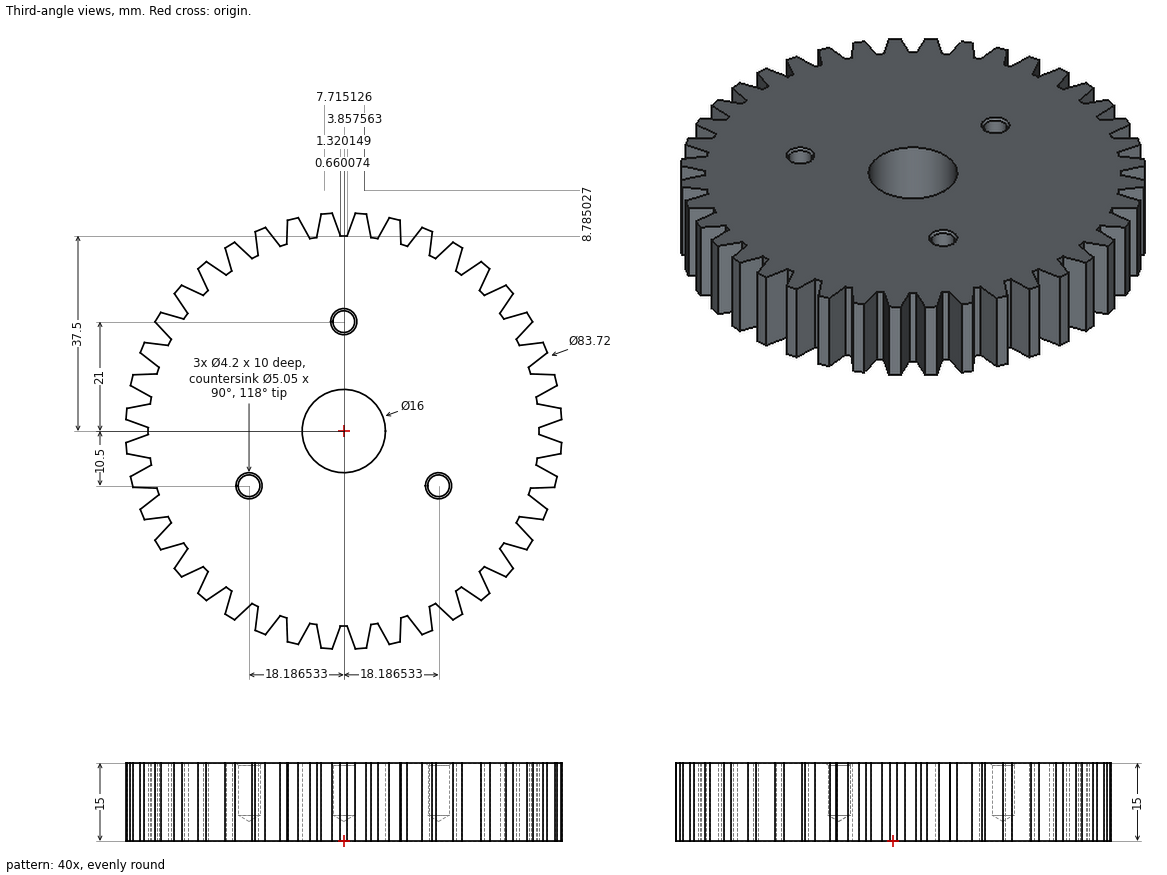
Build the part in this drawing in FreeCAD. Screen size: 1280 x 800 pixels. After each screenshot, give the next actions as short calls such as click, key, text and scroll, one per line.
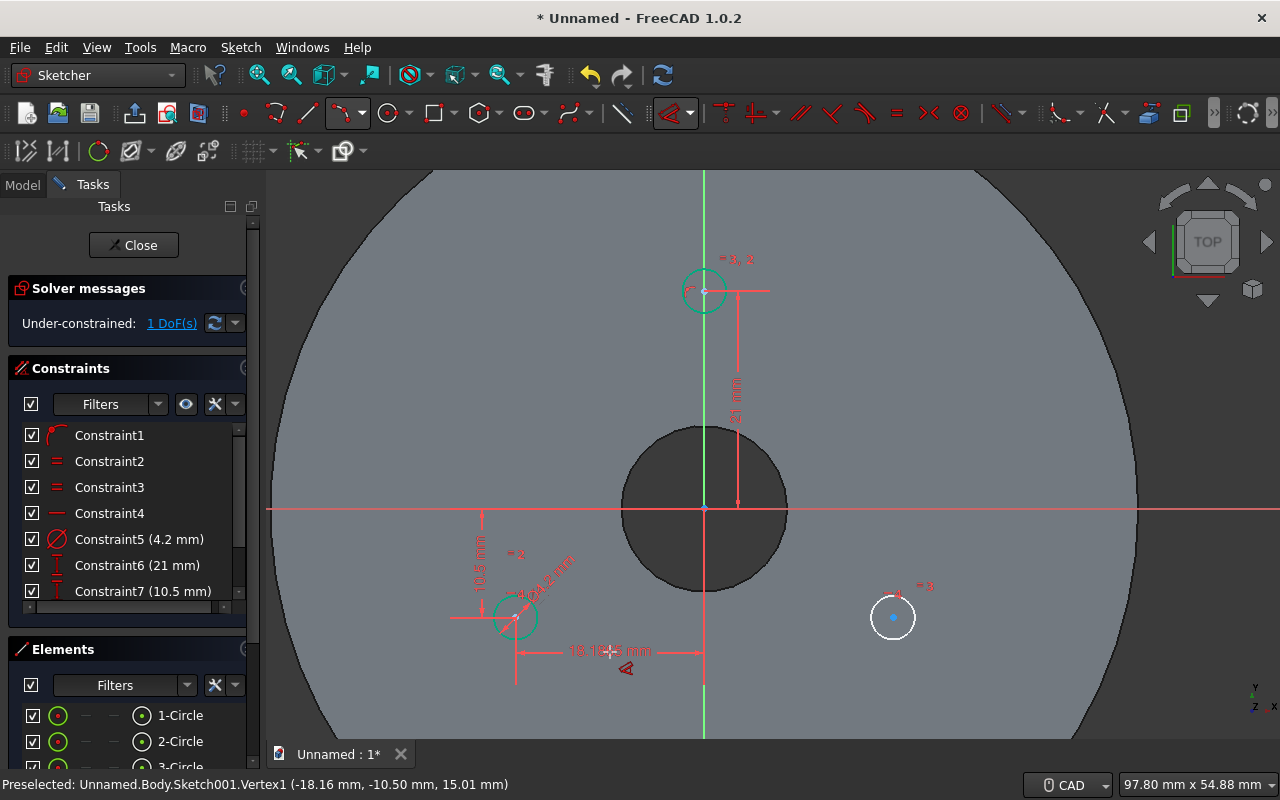
click(893, 618)
click(799, 652)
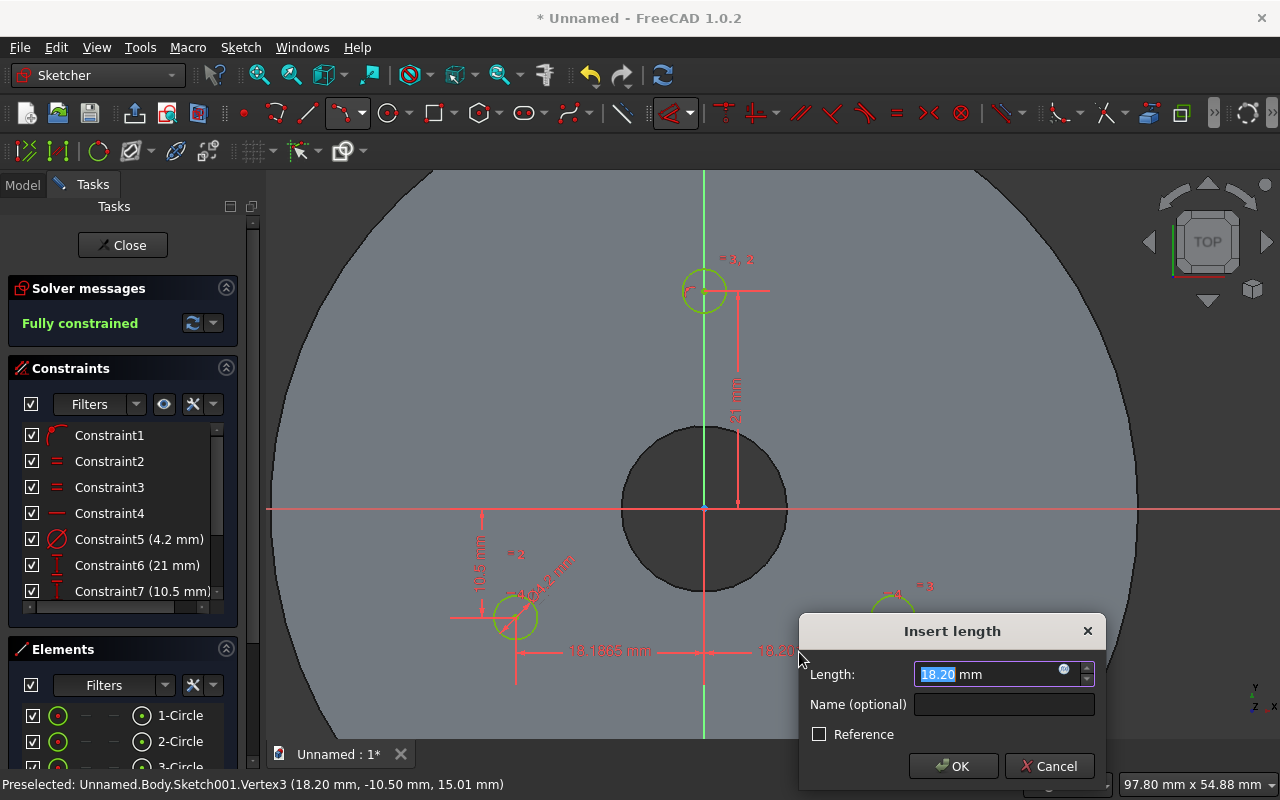
text(18.186533)
key(Return)
key(Escape)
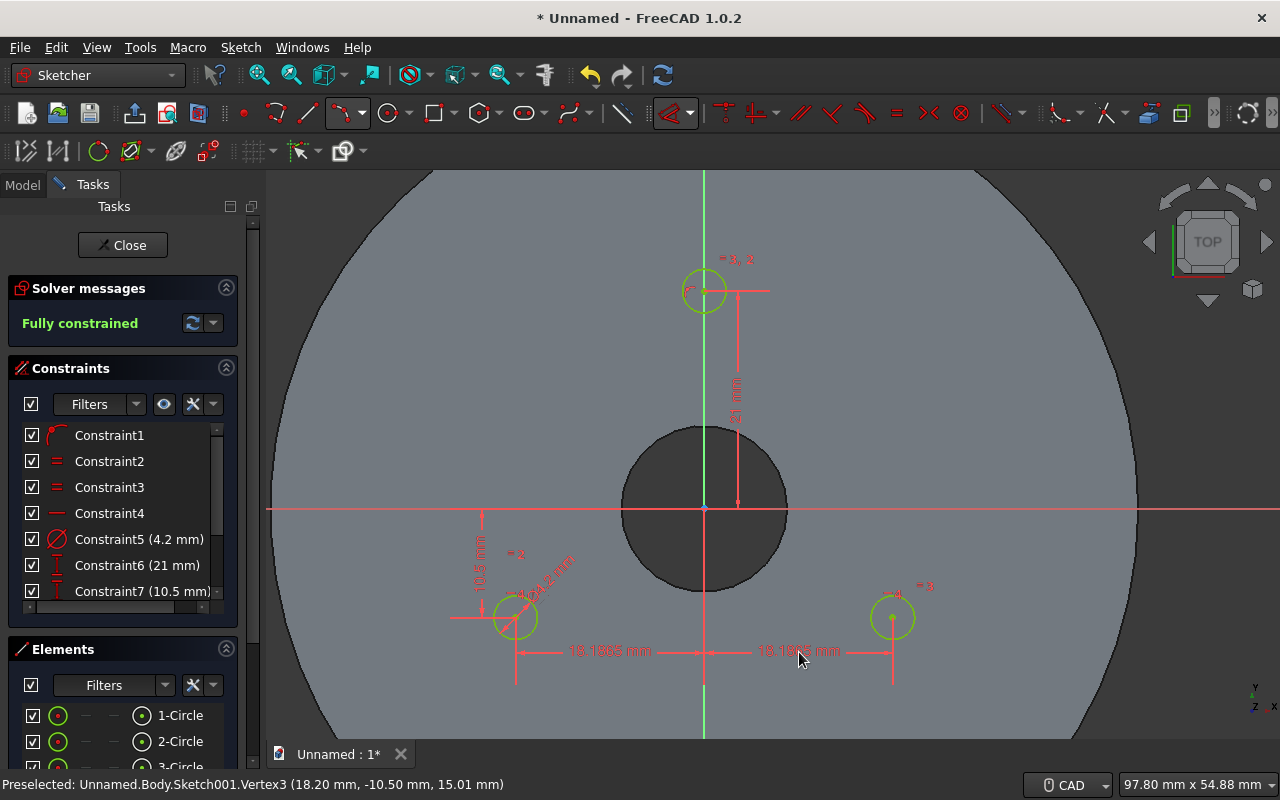
click(123, 245)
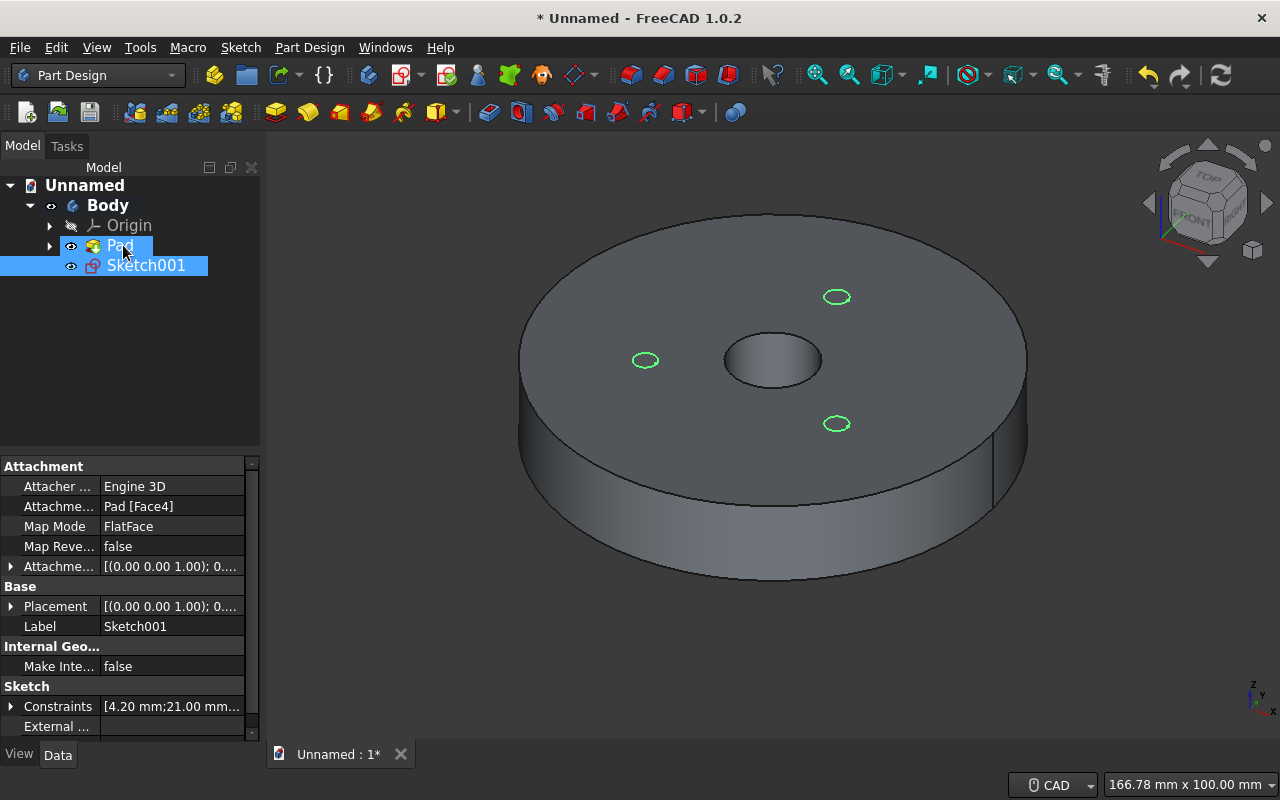
click(522, 112)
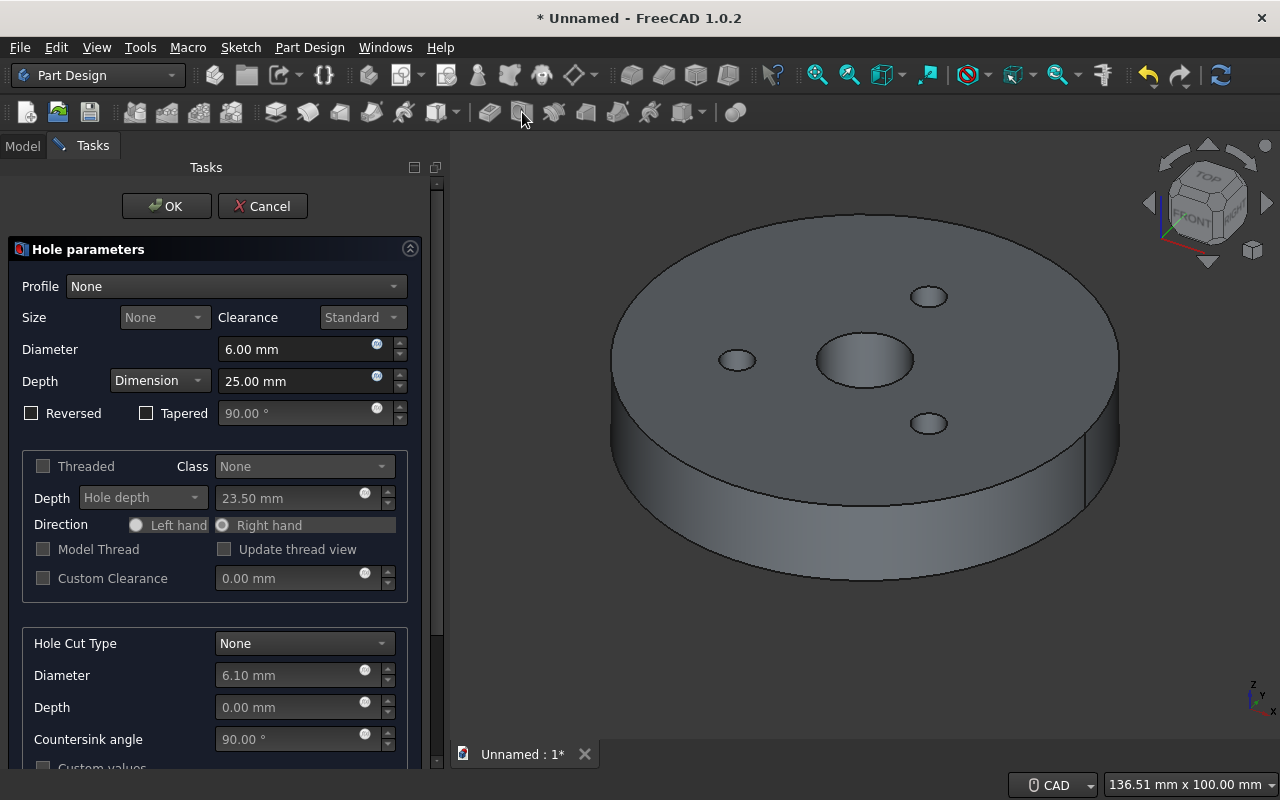
triple_click(305, 349)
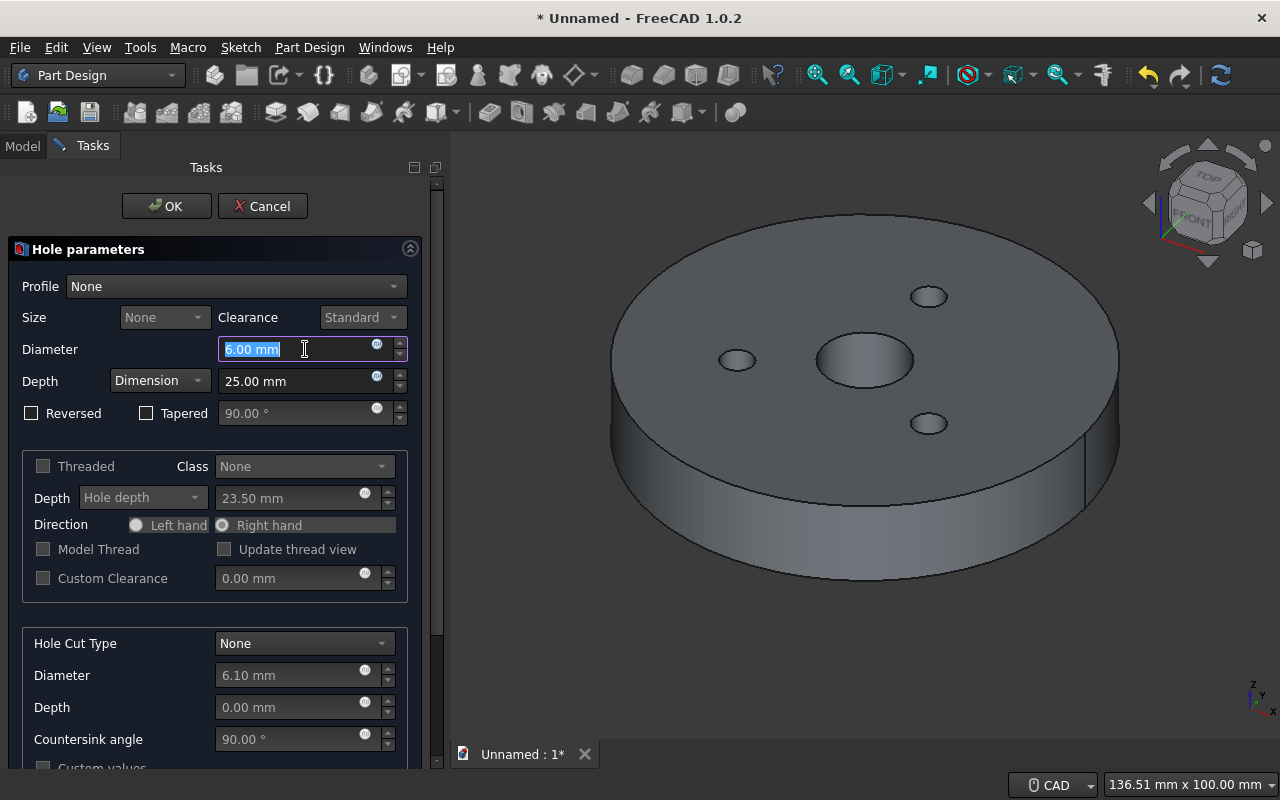
text(4.2)
key(Tab)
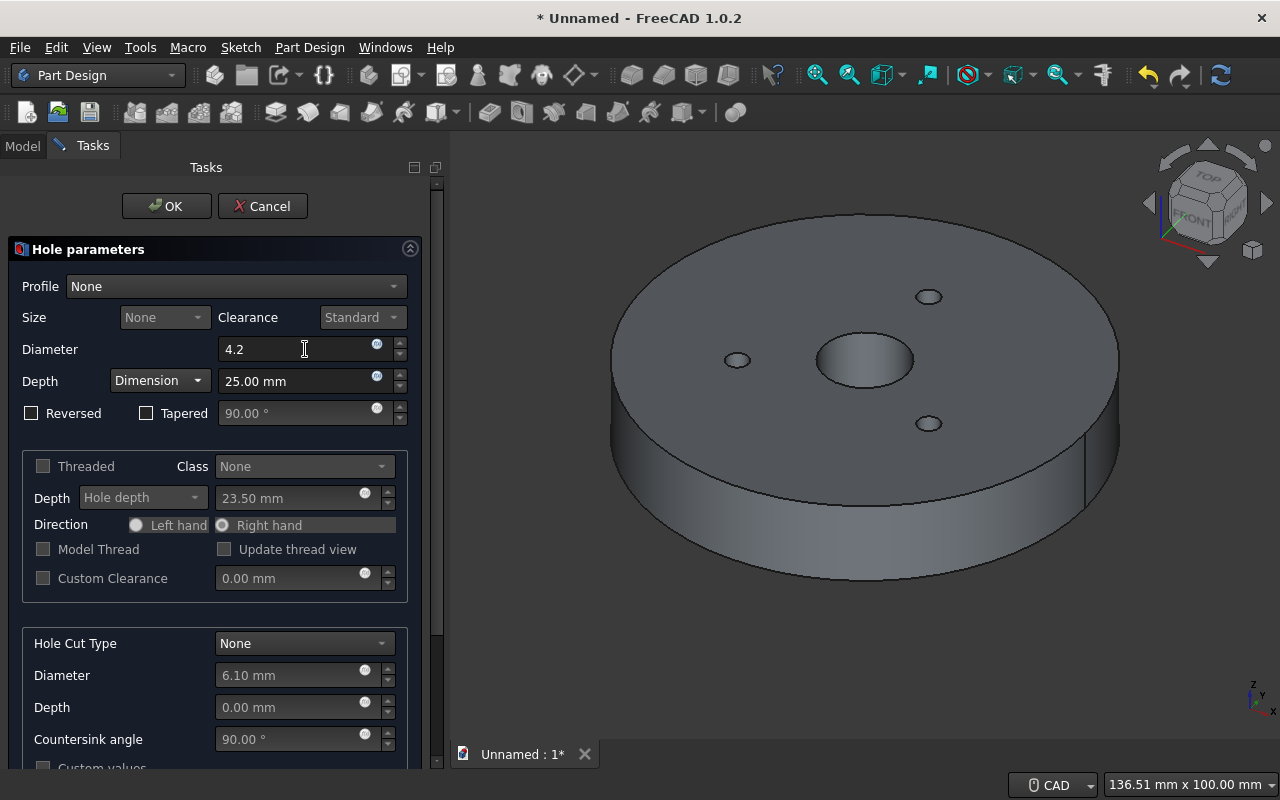
triple_click(305, 381)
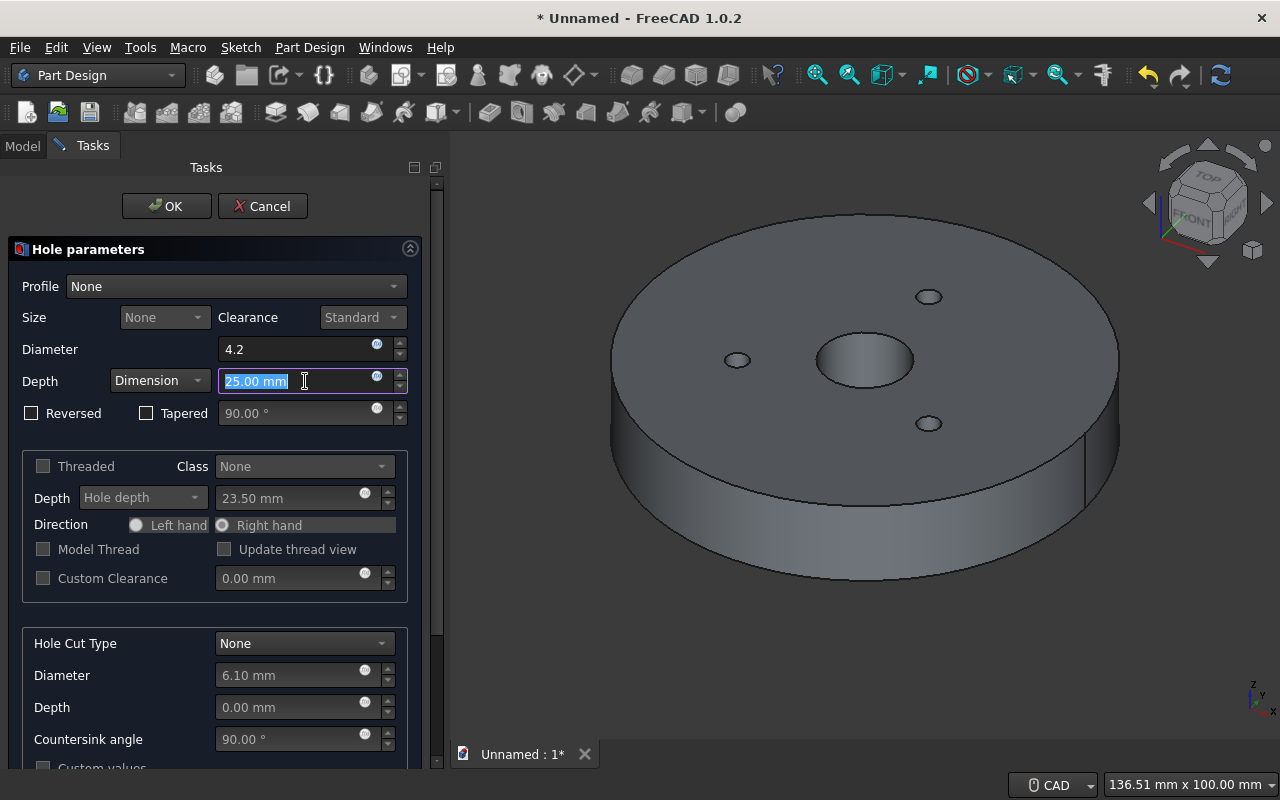
text(10)
key(Tab)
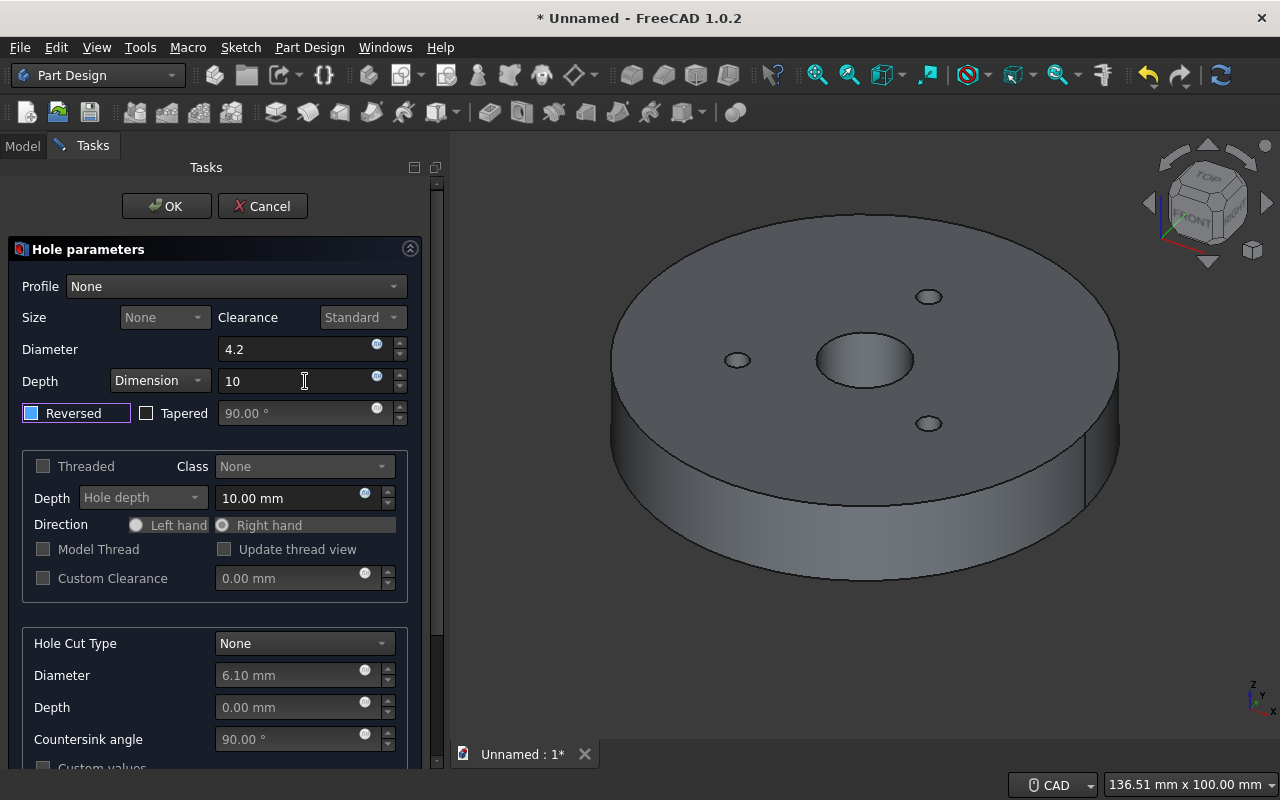
click(306, 644)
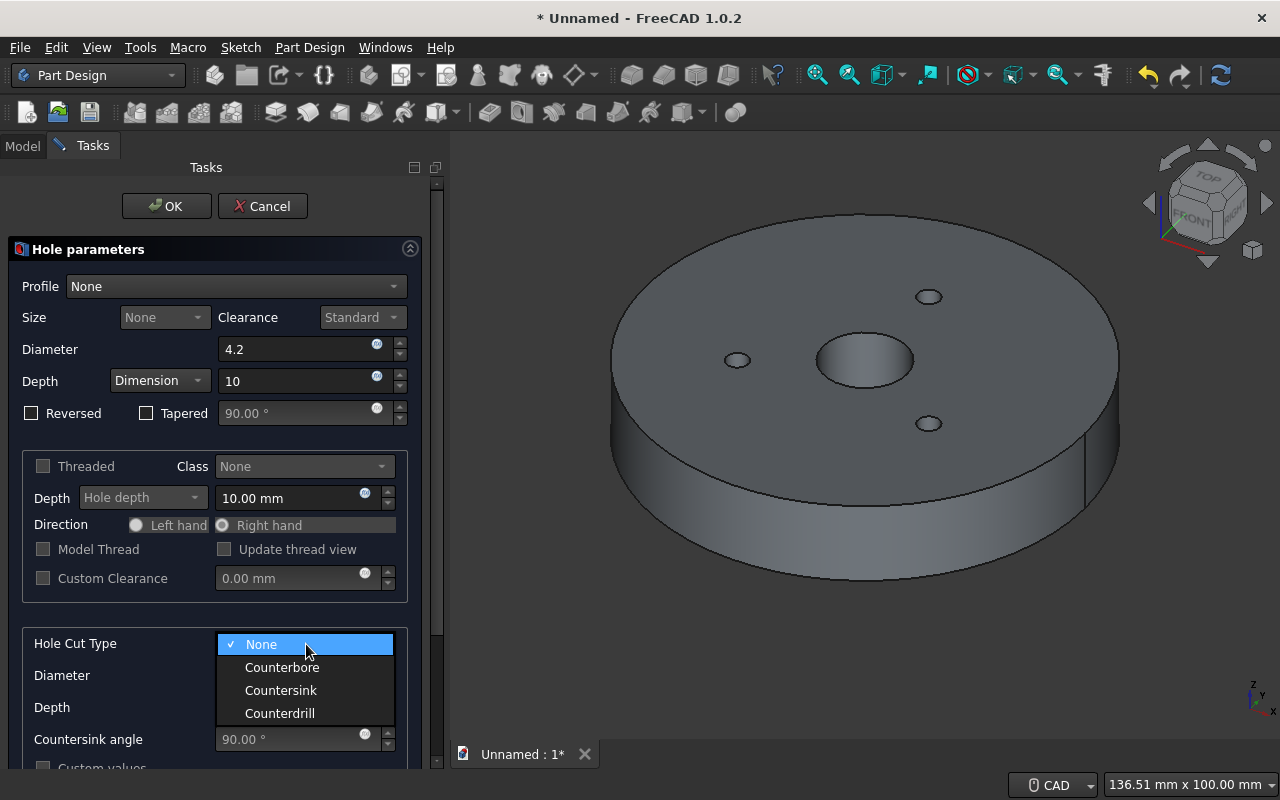
click(304, 690)